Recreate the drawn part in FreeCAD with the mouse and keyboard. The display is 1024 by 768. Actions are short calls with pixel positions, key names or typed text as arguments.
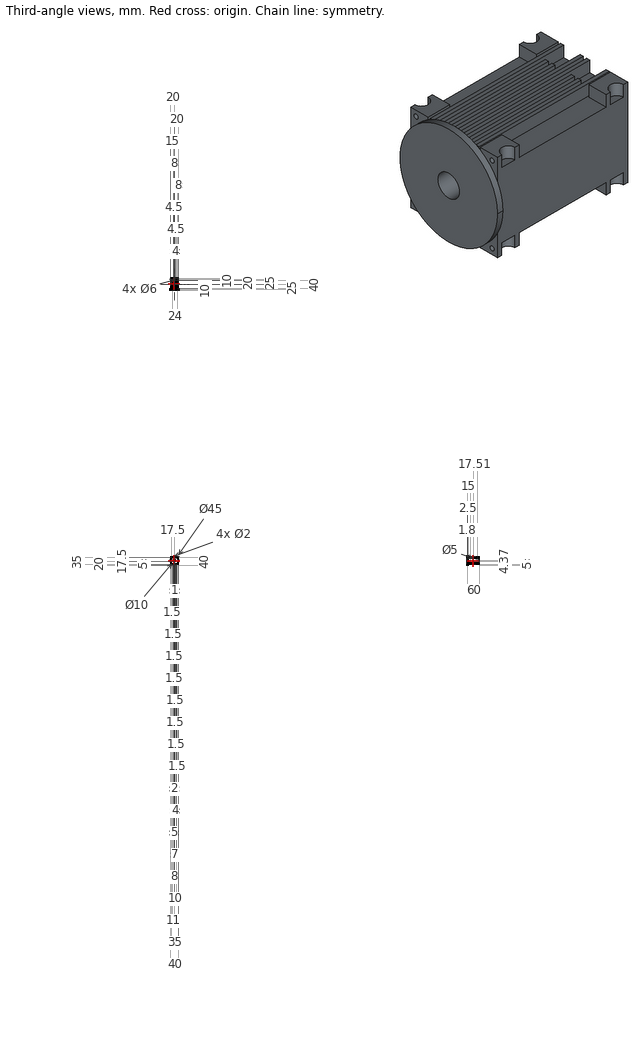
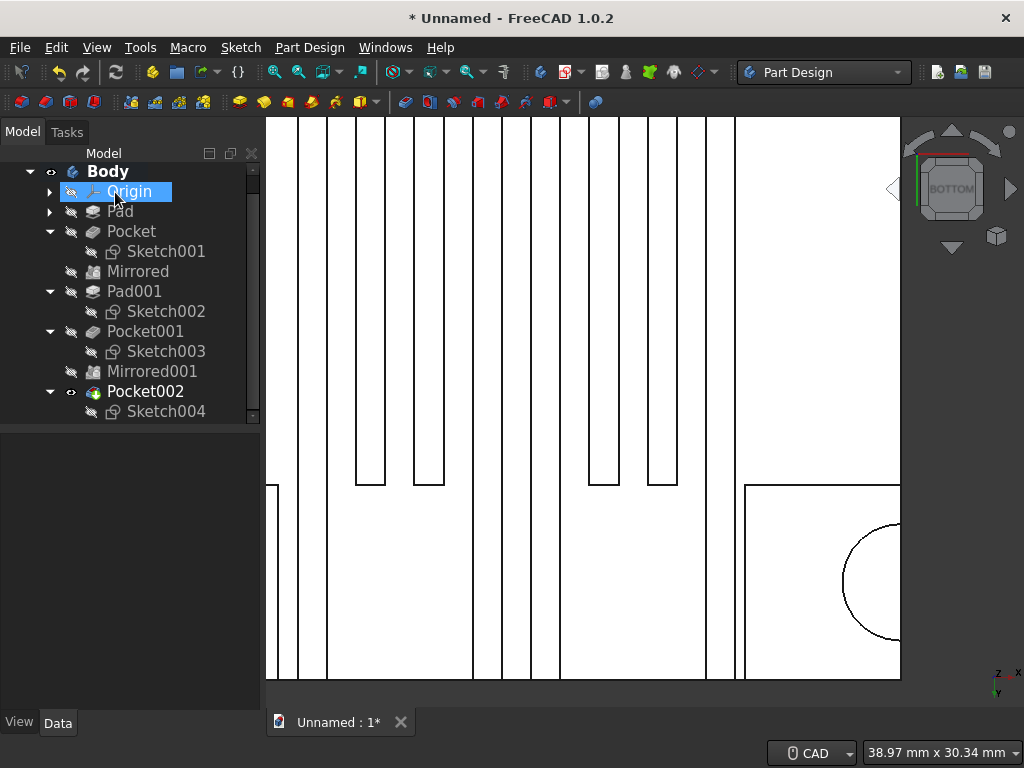
click(276, 72)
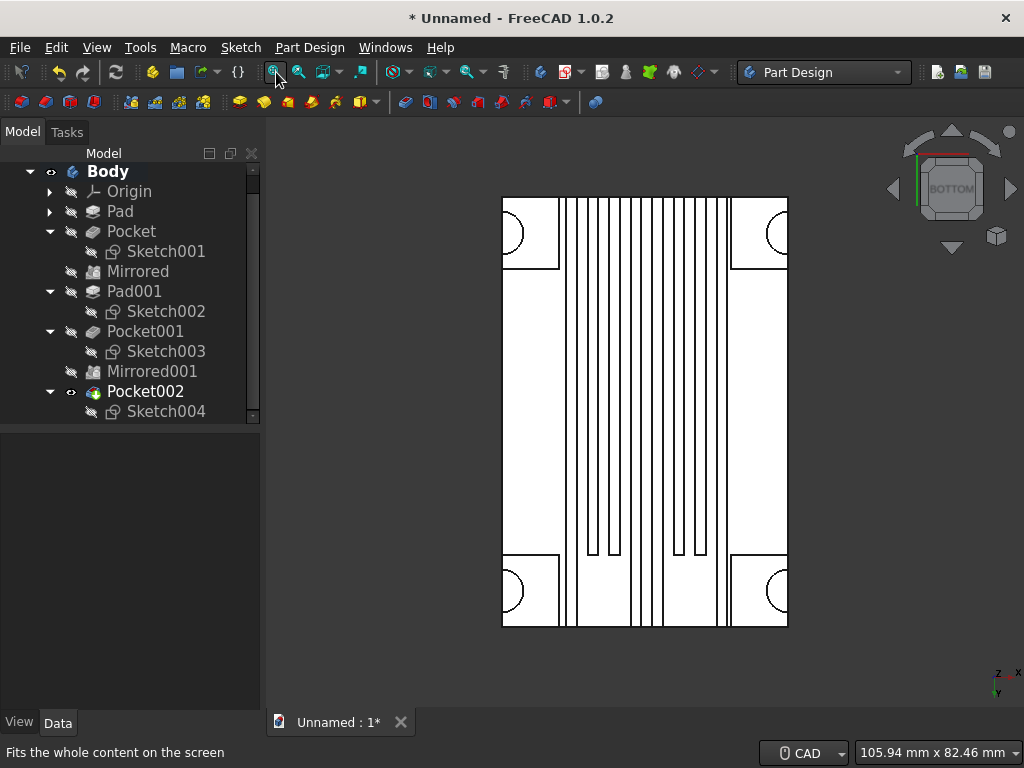
click(116, 392)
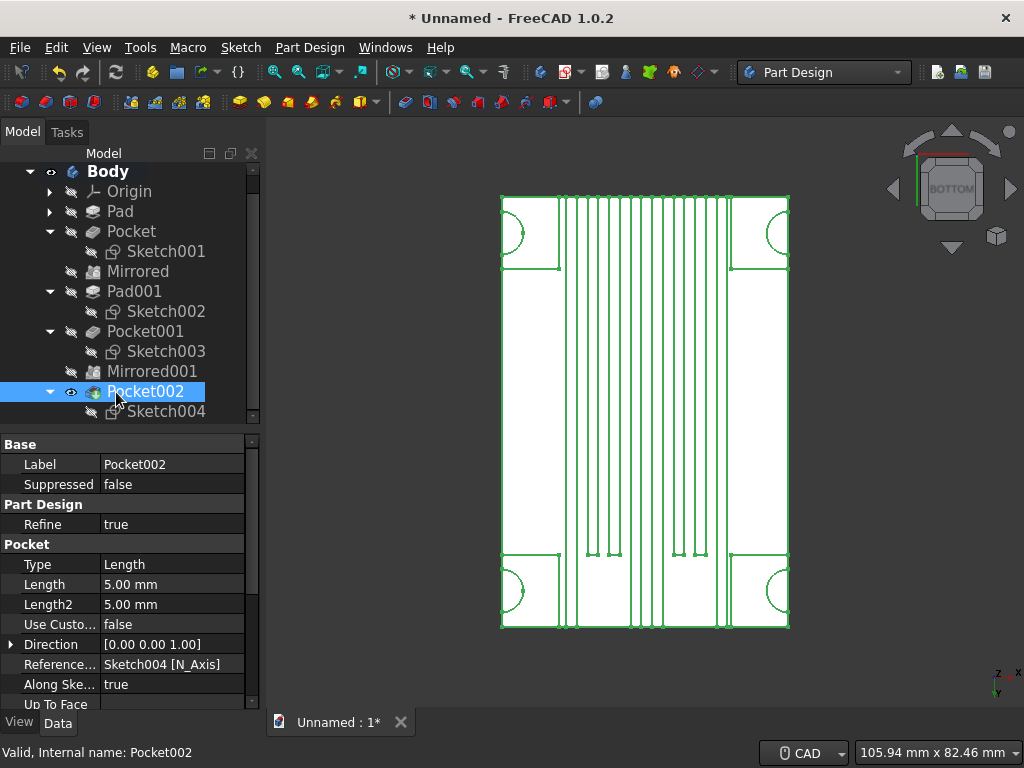
click(132, 102)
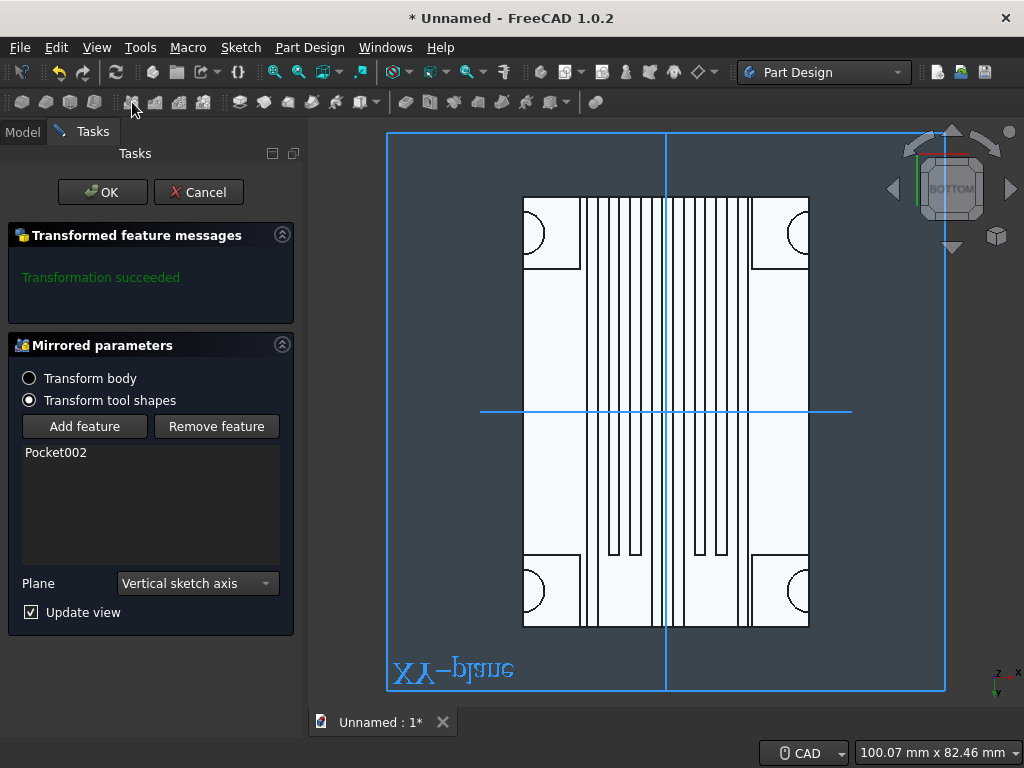
click(198, 584)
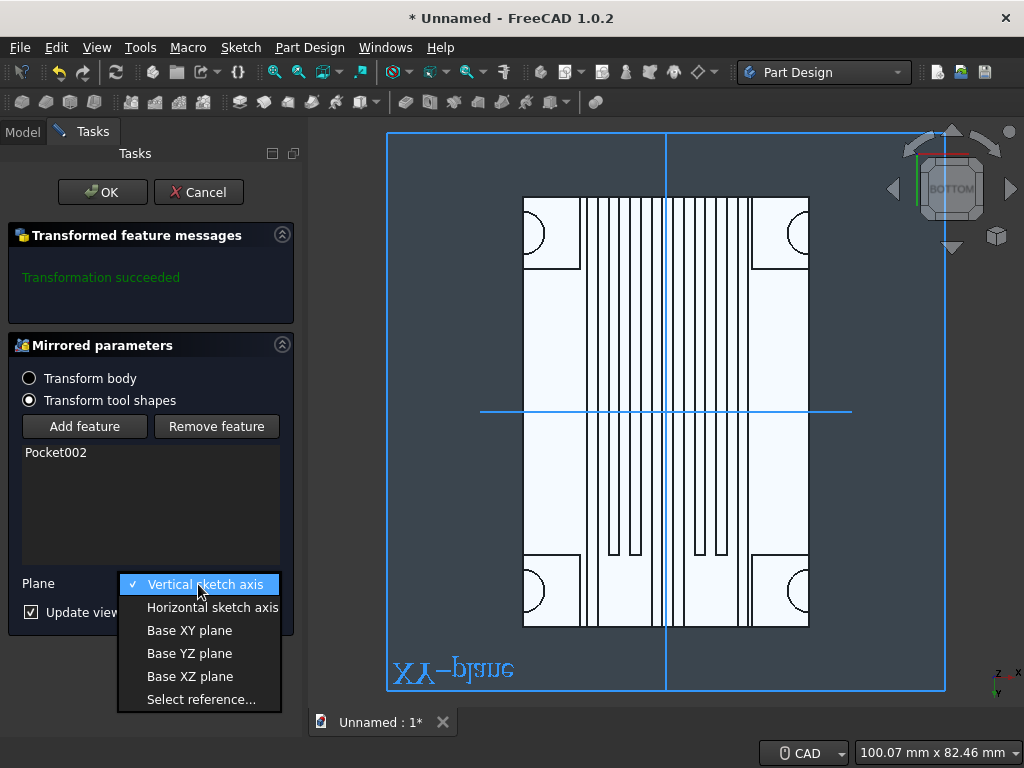
click(198, 630)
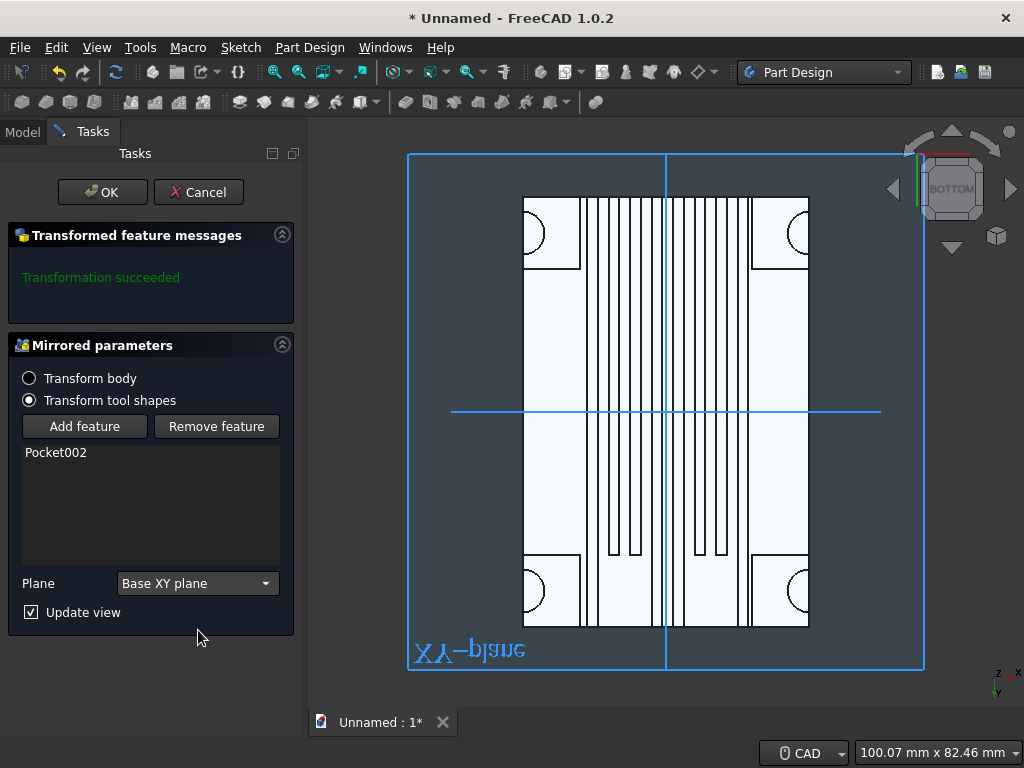
click(103, 192)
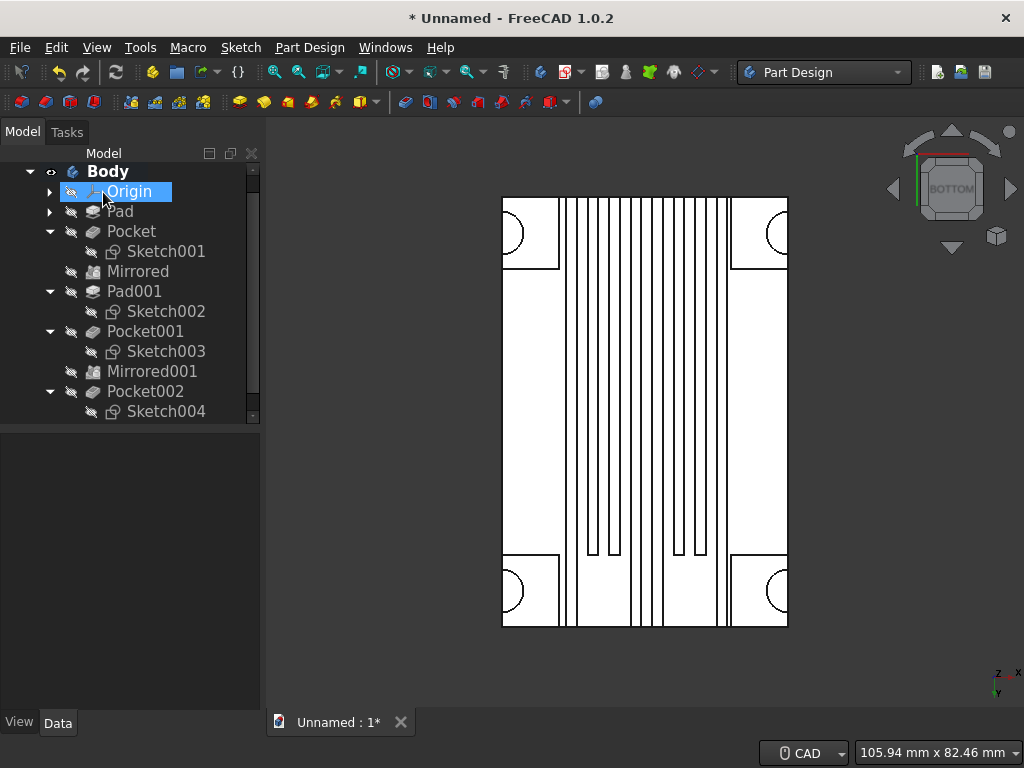
key(0)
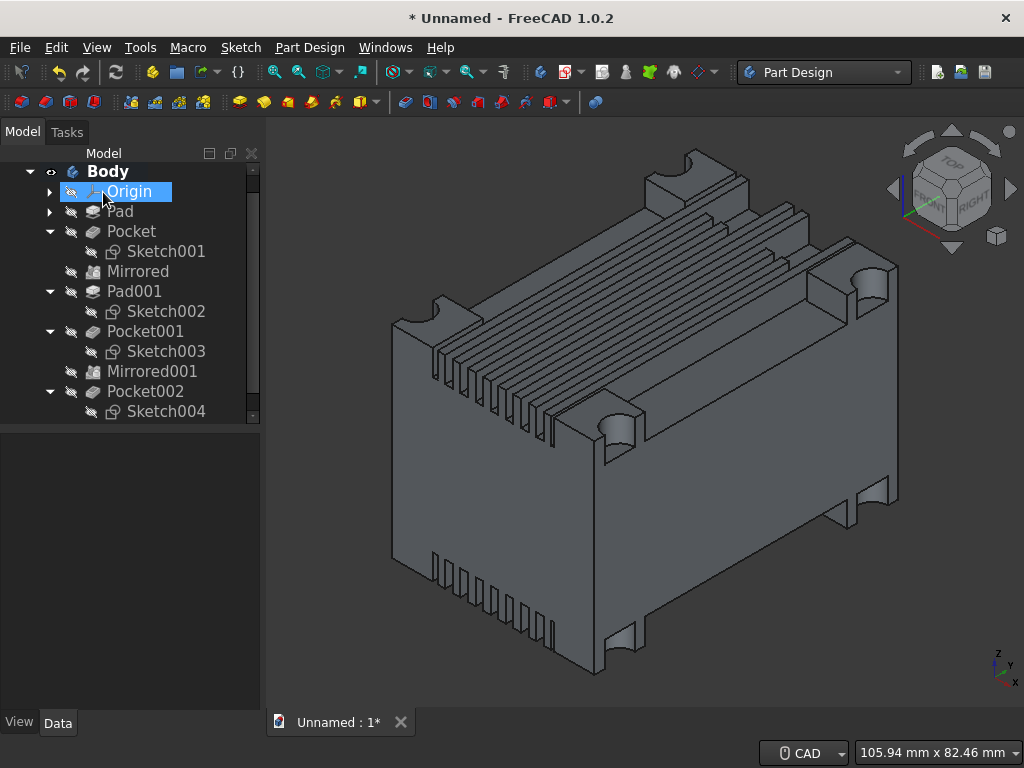
click(493, 499)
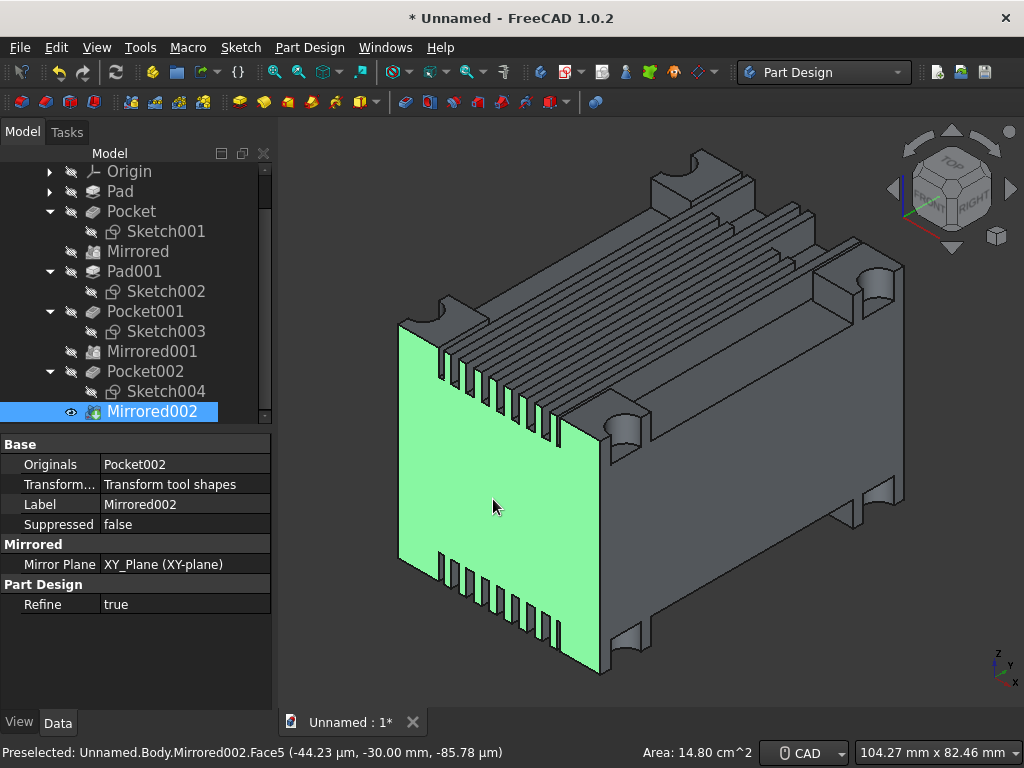
click(566, 72)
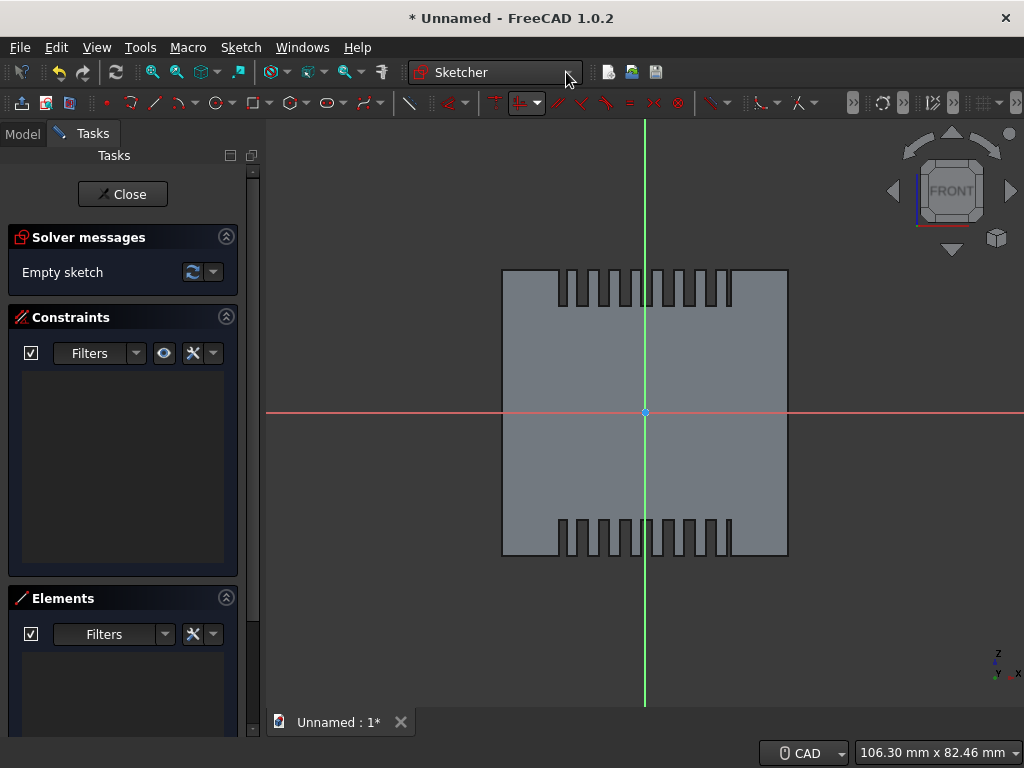
key(g)
key(c)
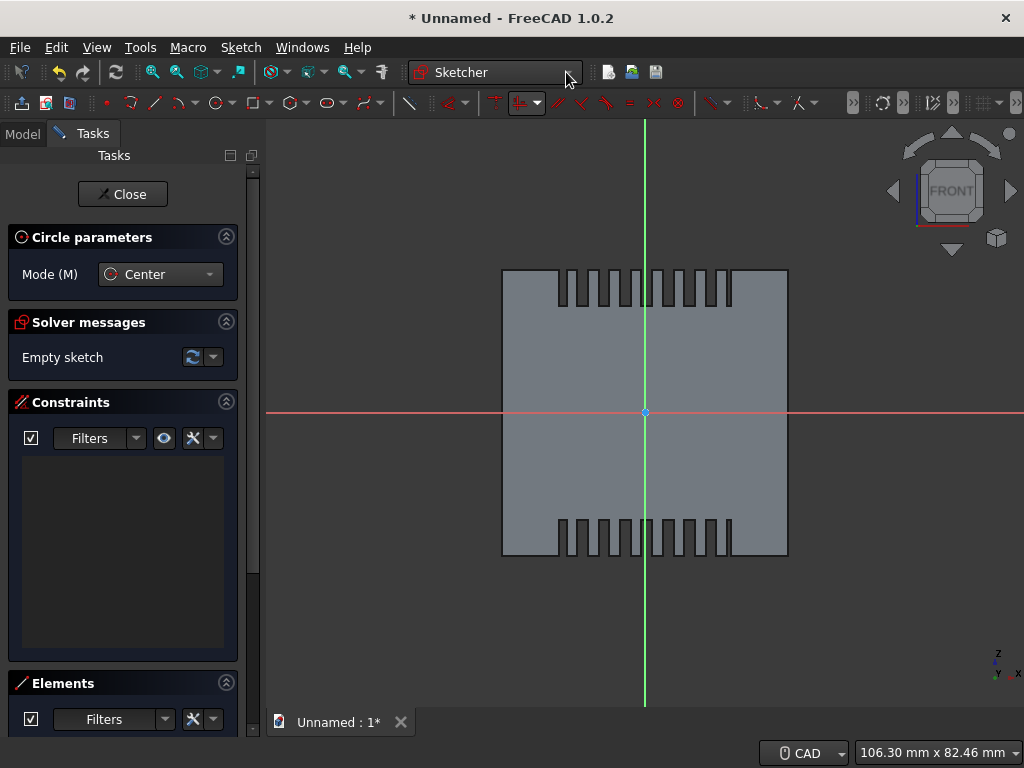
click(645, 413)
click(758, 300)
key(Escape)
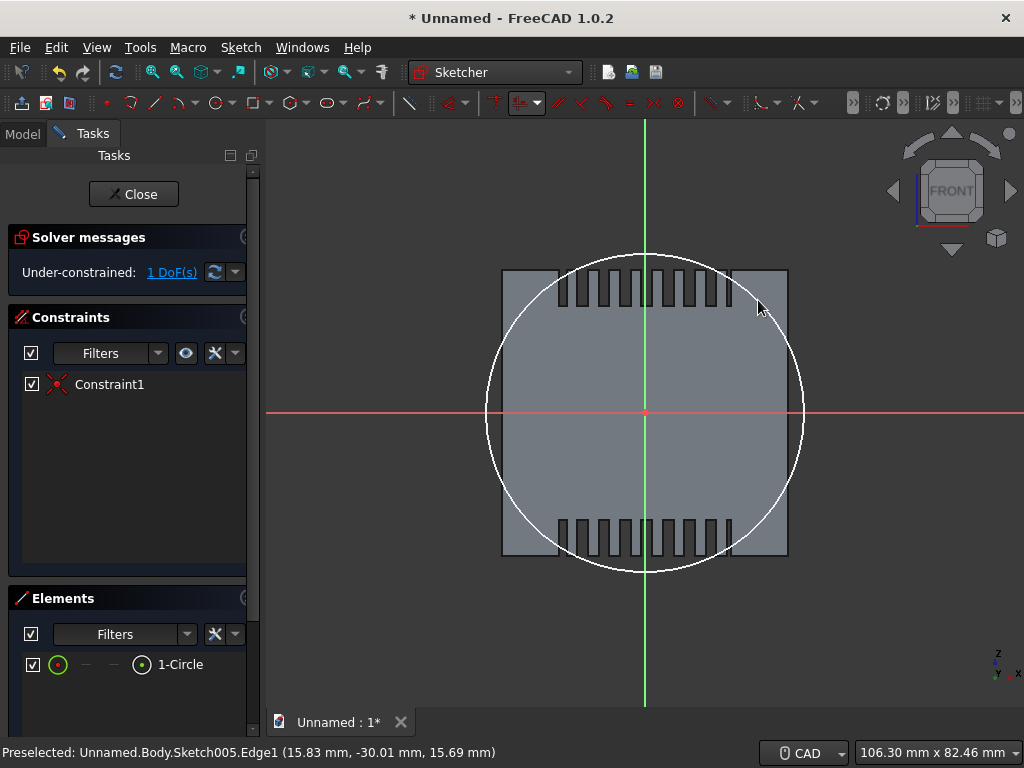
click(448, 104)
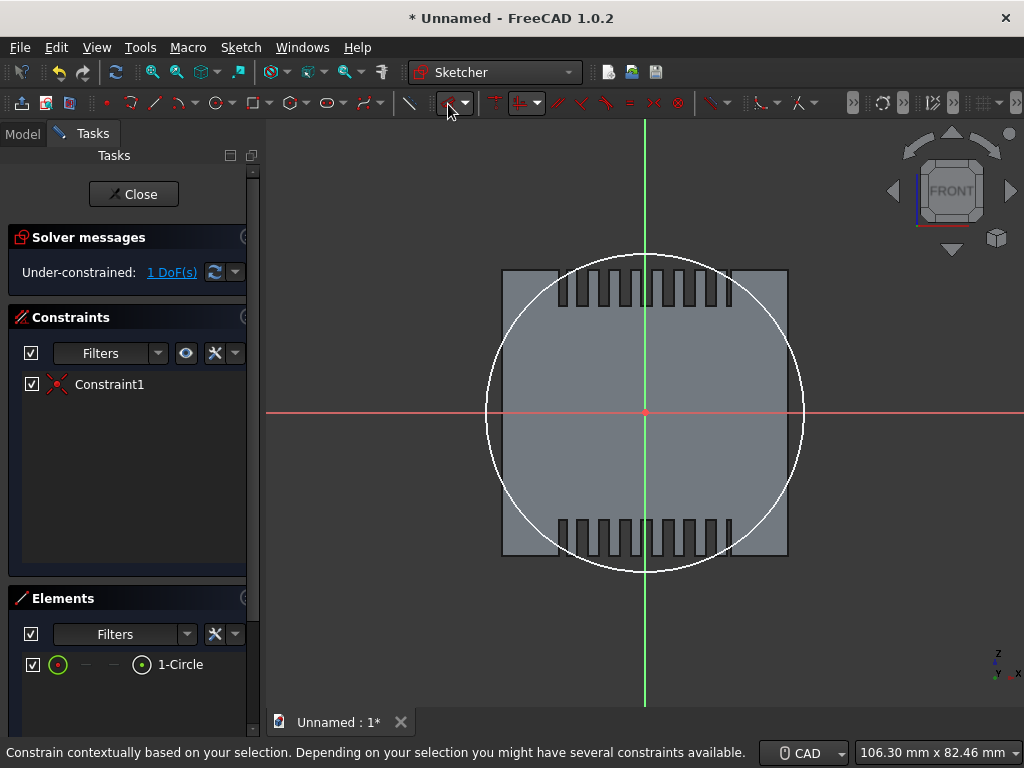
click(757, 300)
click(780, 277)